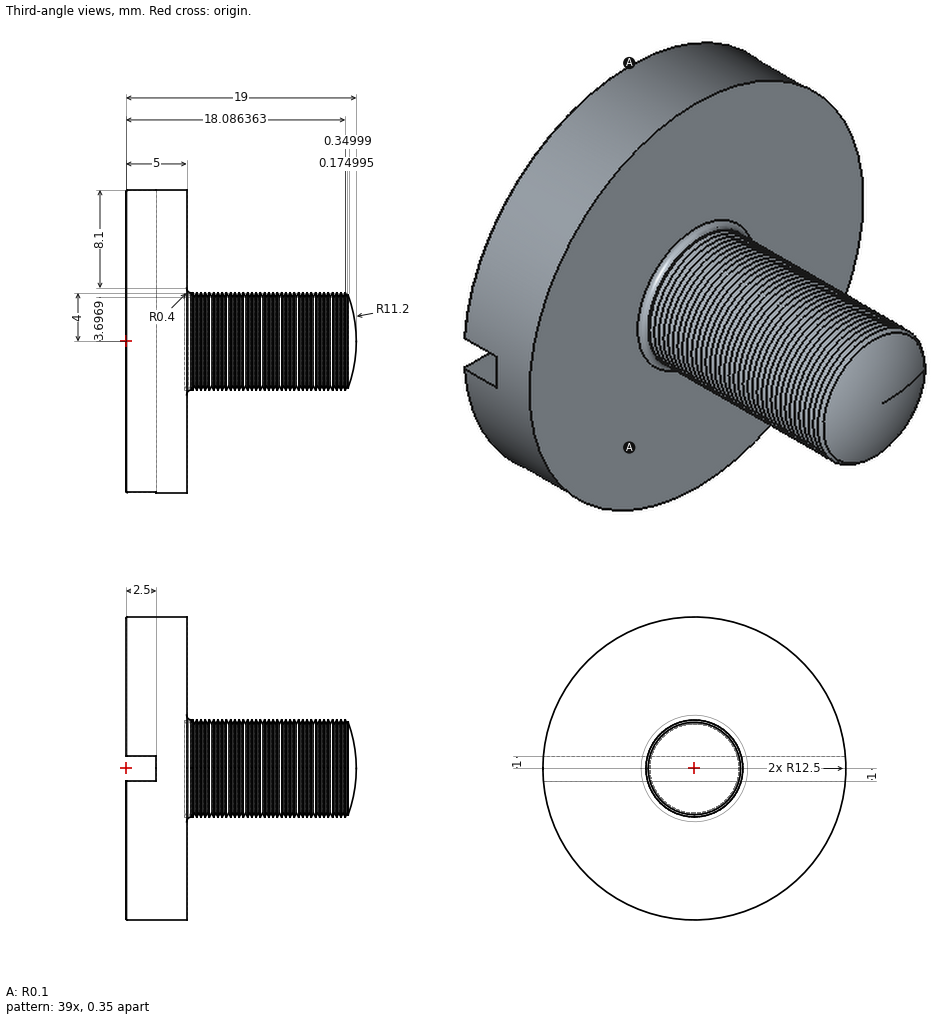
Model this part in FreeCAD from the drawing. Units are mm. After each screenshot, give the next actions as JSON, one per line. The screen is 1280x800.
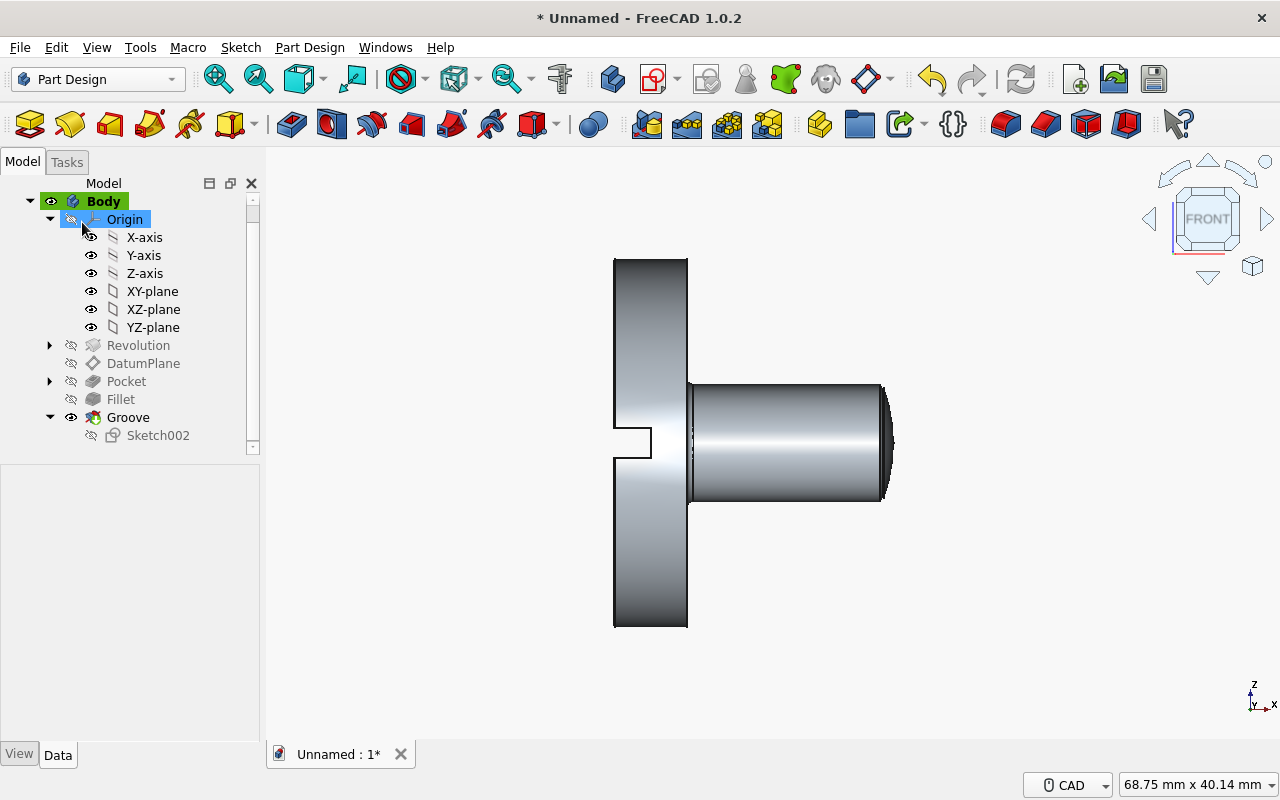
{"action": "left_click", "coordinate": [116, 417]}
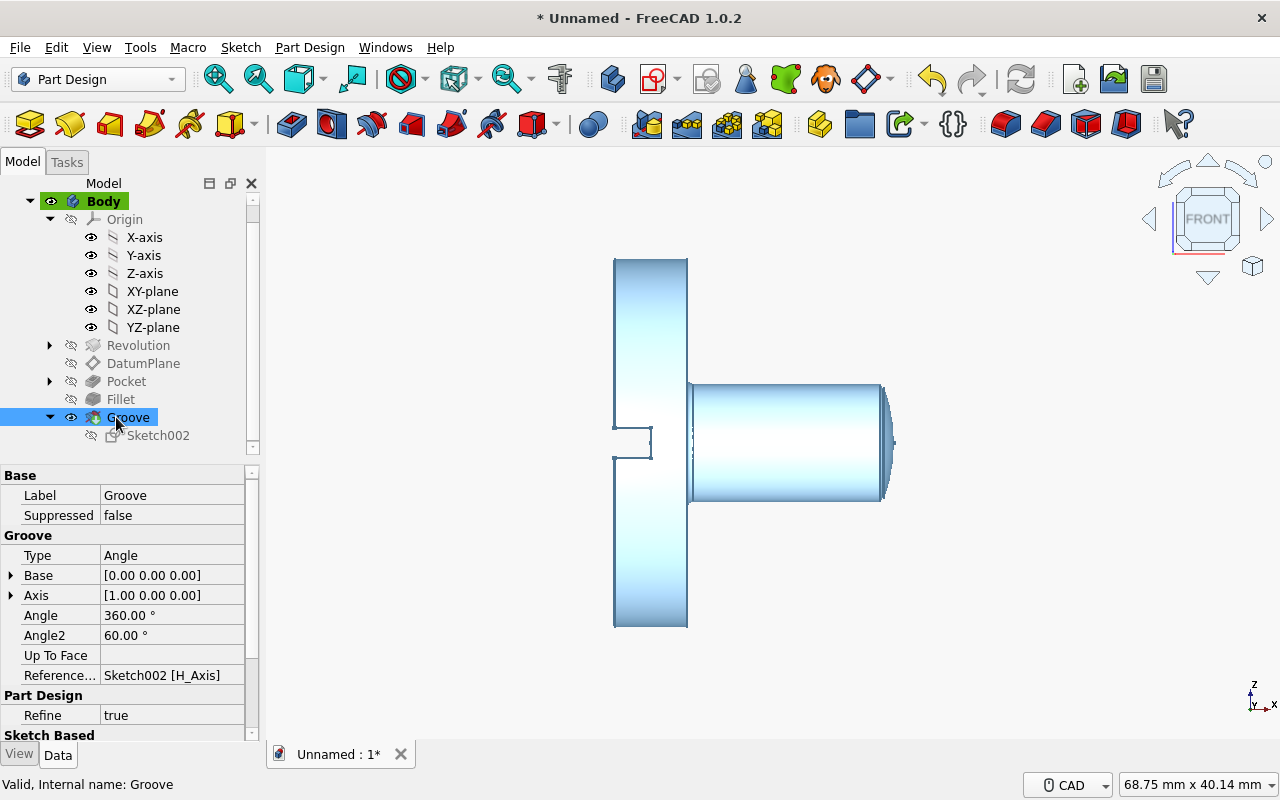
{"action": "left_click", "coordinate": [688, 124]}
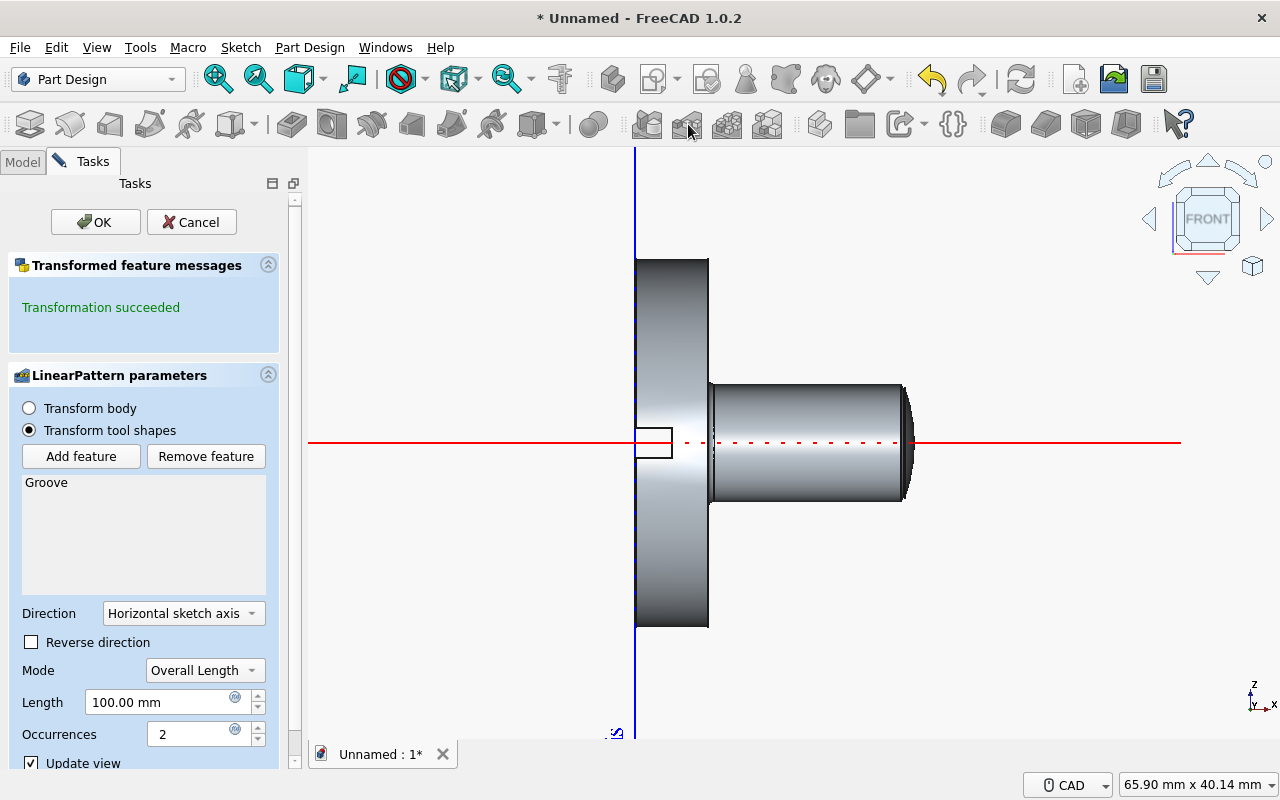
{"action": "left_click", "coordinate": [184, 614]}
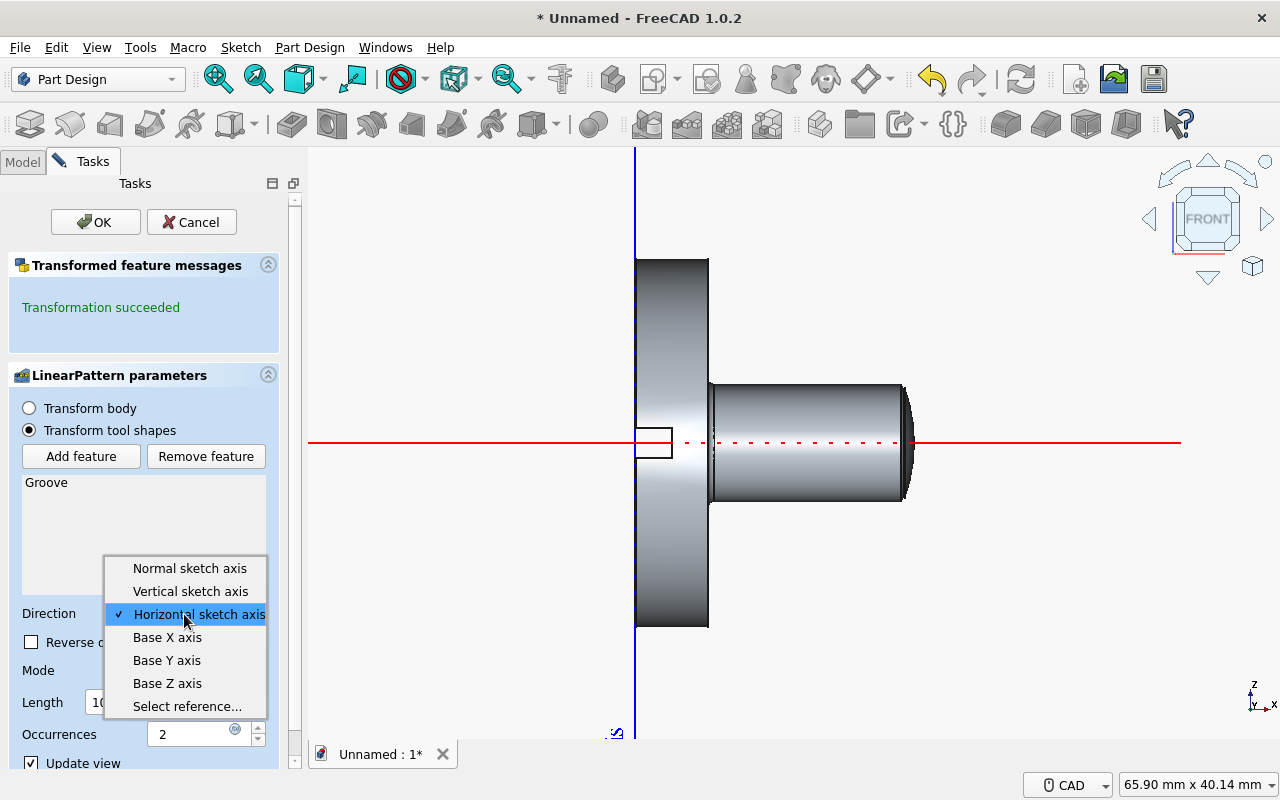
{"action": "left_click", "coordinate": [184, 638]}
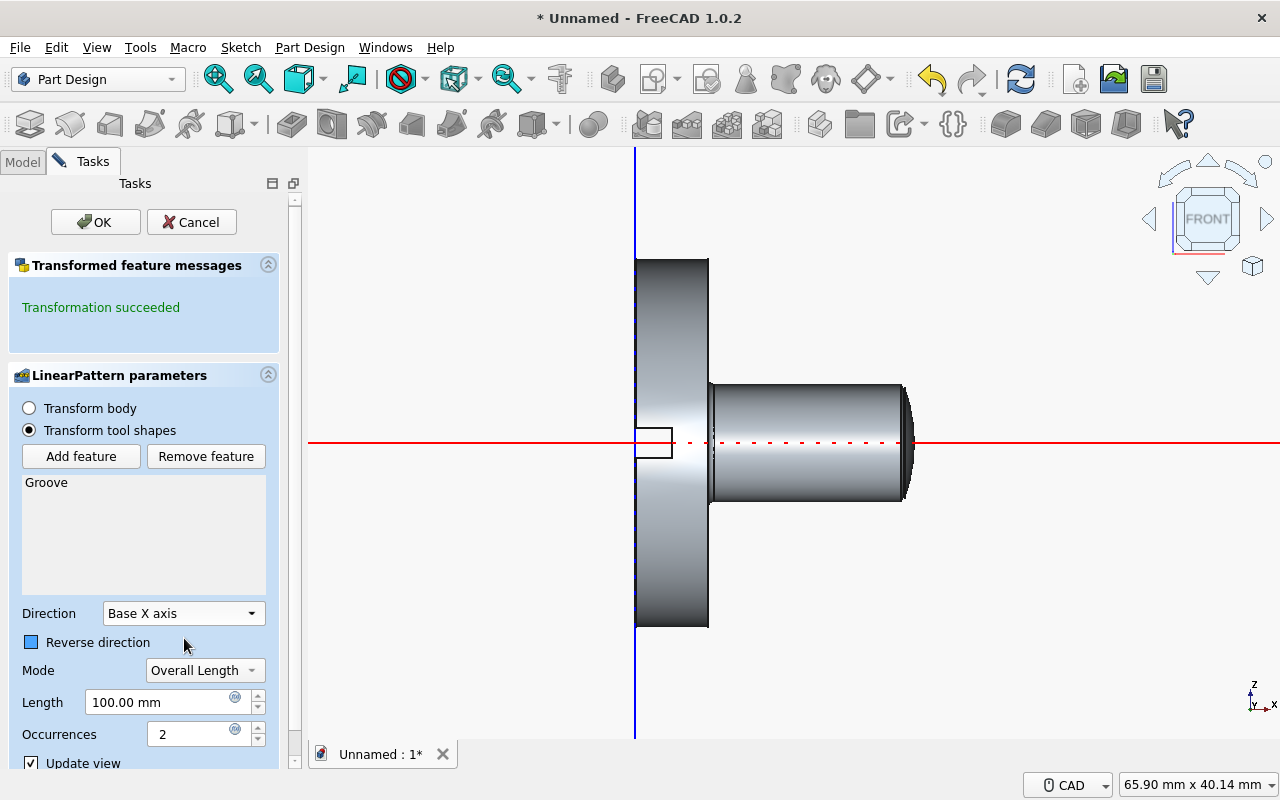
{"action": "left_click", "coordinate": [206, 670]}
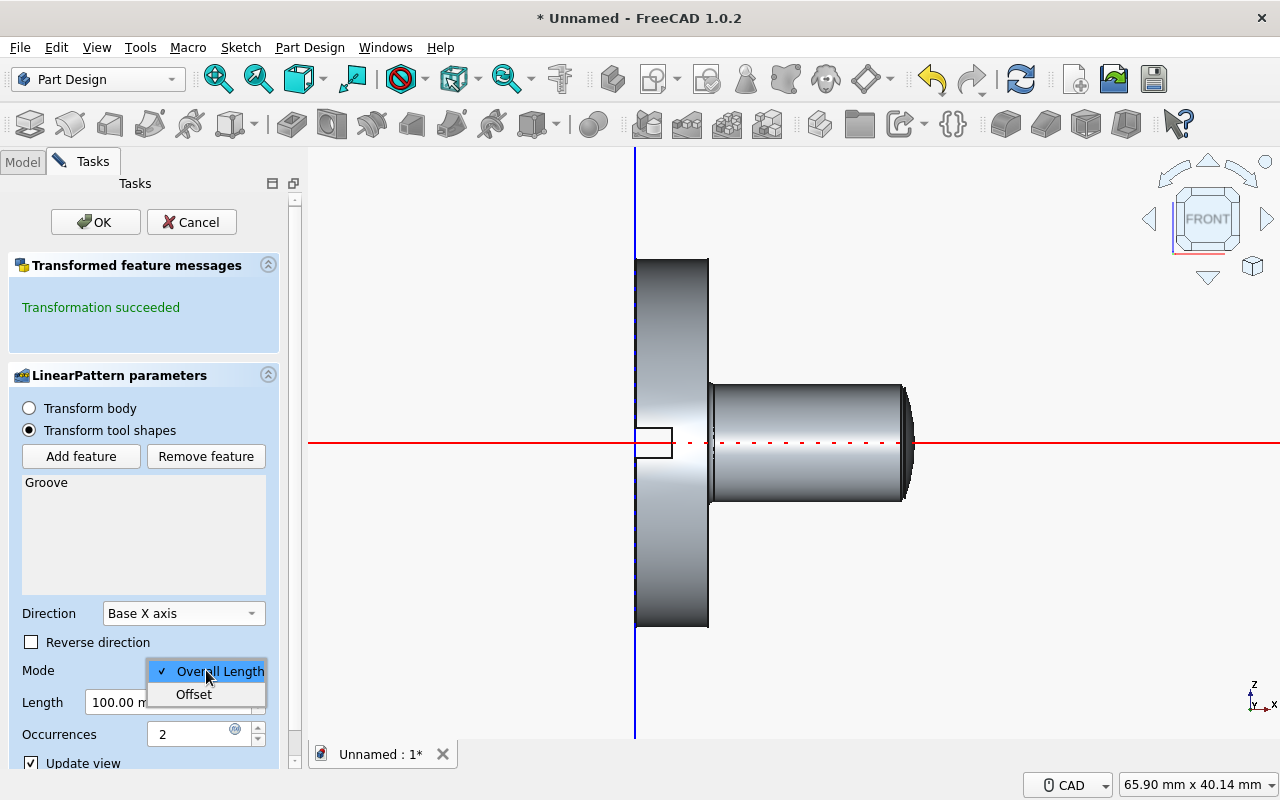
{"action": "left_click", "coordinate": [206, 694]}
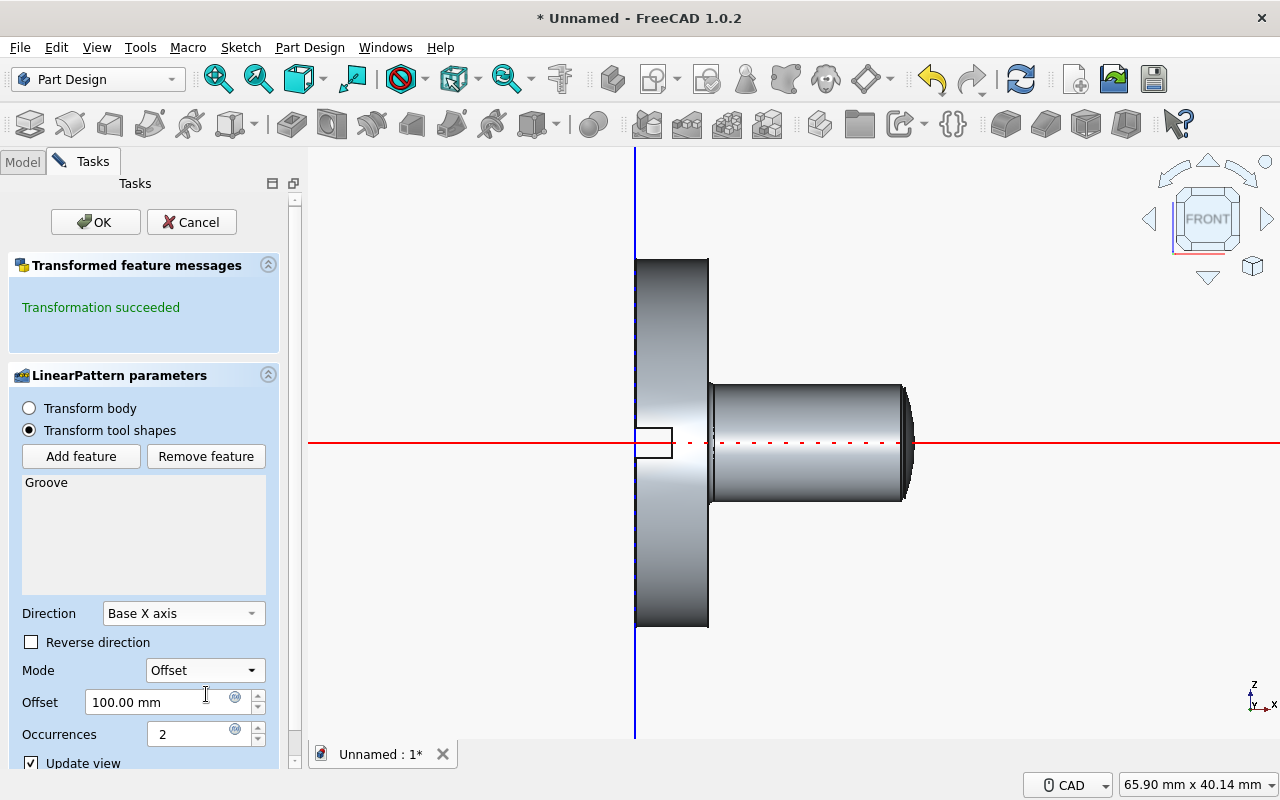
{"action": "triple_click", "coordinate": [168, 702]}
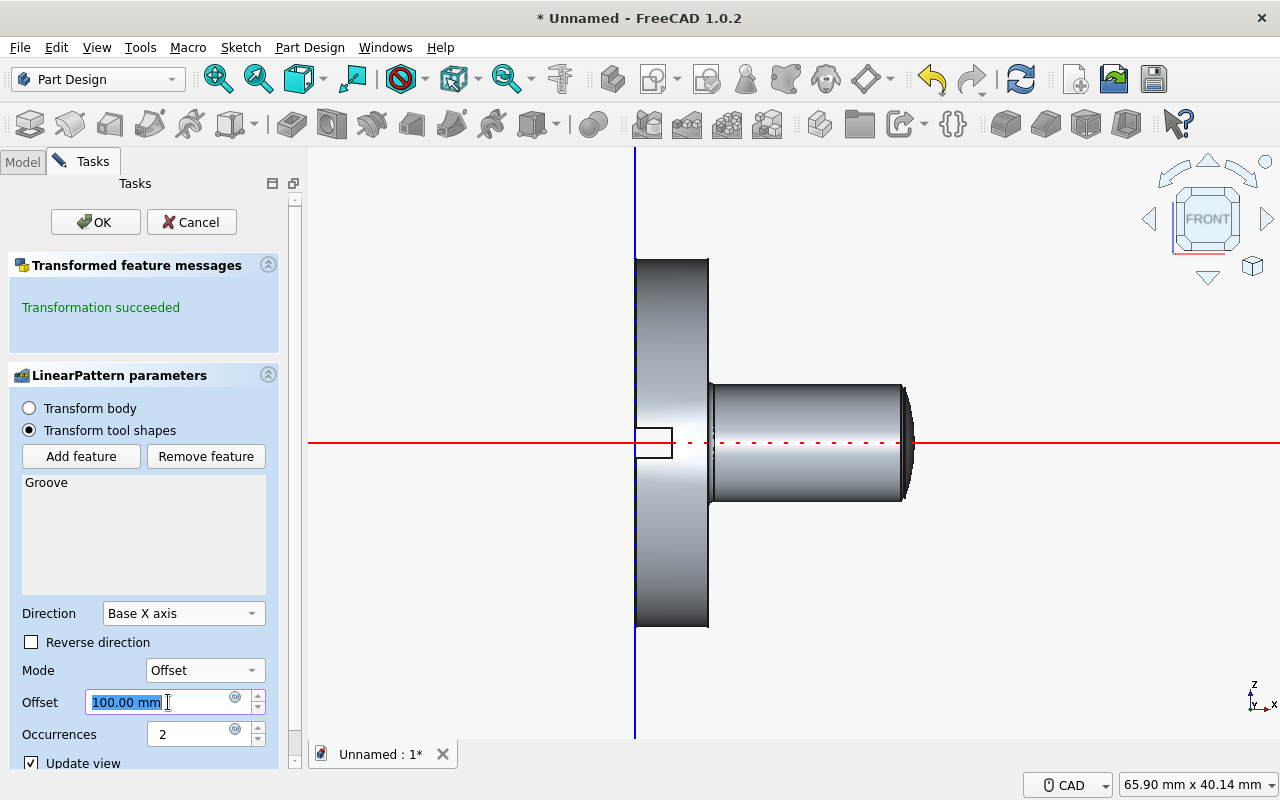
{"action": "type", "text": "0.35"}
{"action": "key", "text": "Tab"}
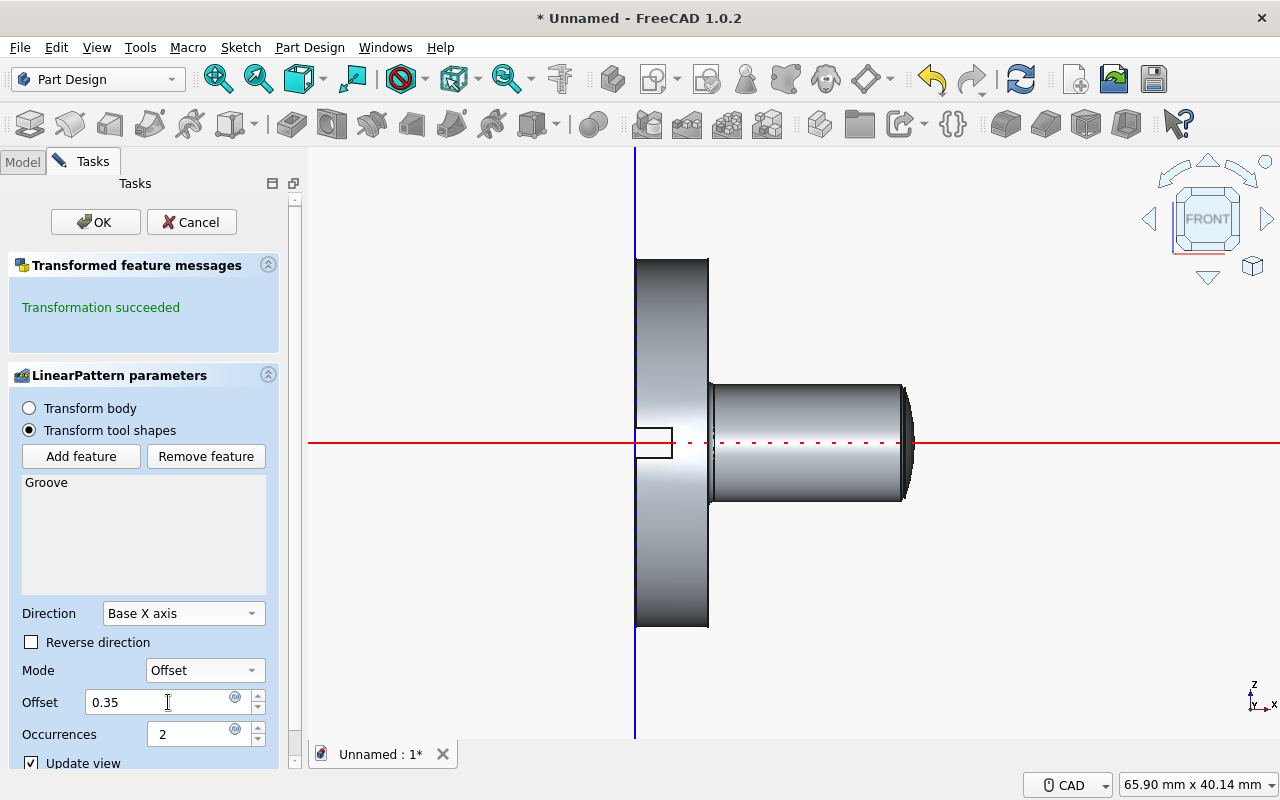
{"action": "triple_click", "coordinate": [198, 734]}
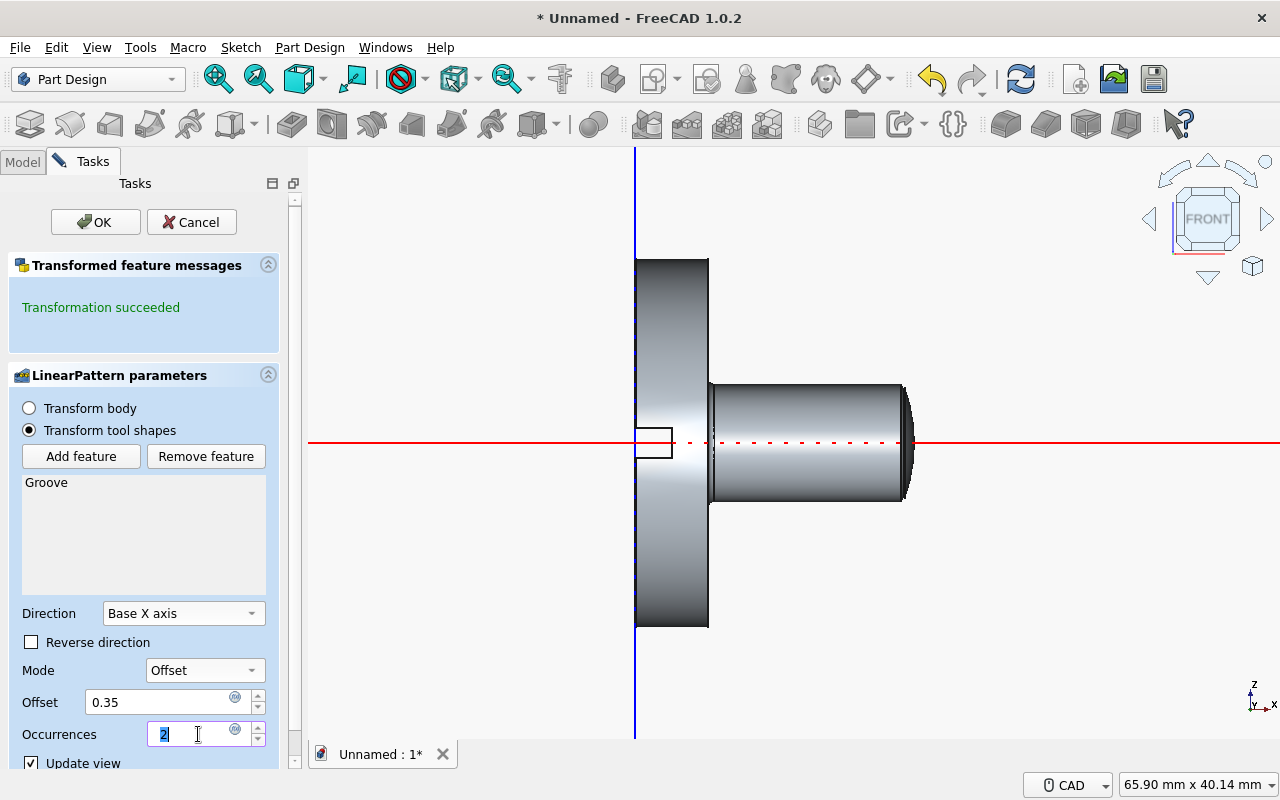
{"action": "type", "text": "39"}
{"action": "key", "text": "Tab"}